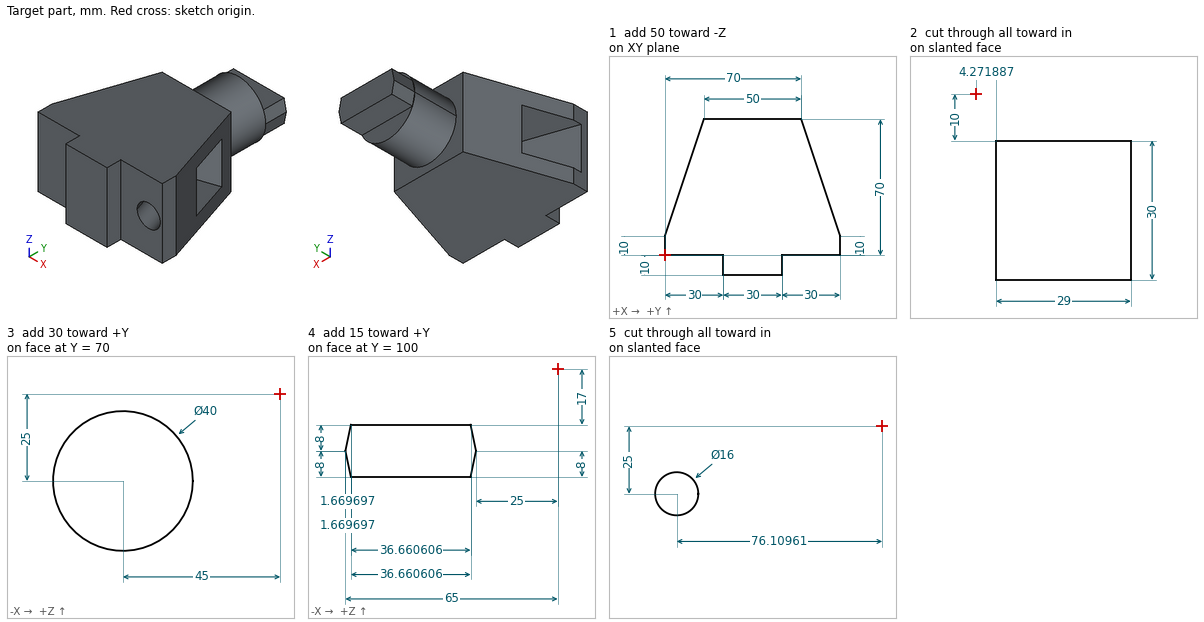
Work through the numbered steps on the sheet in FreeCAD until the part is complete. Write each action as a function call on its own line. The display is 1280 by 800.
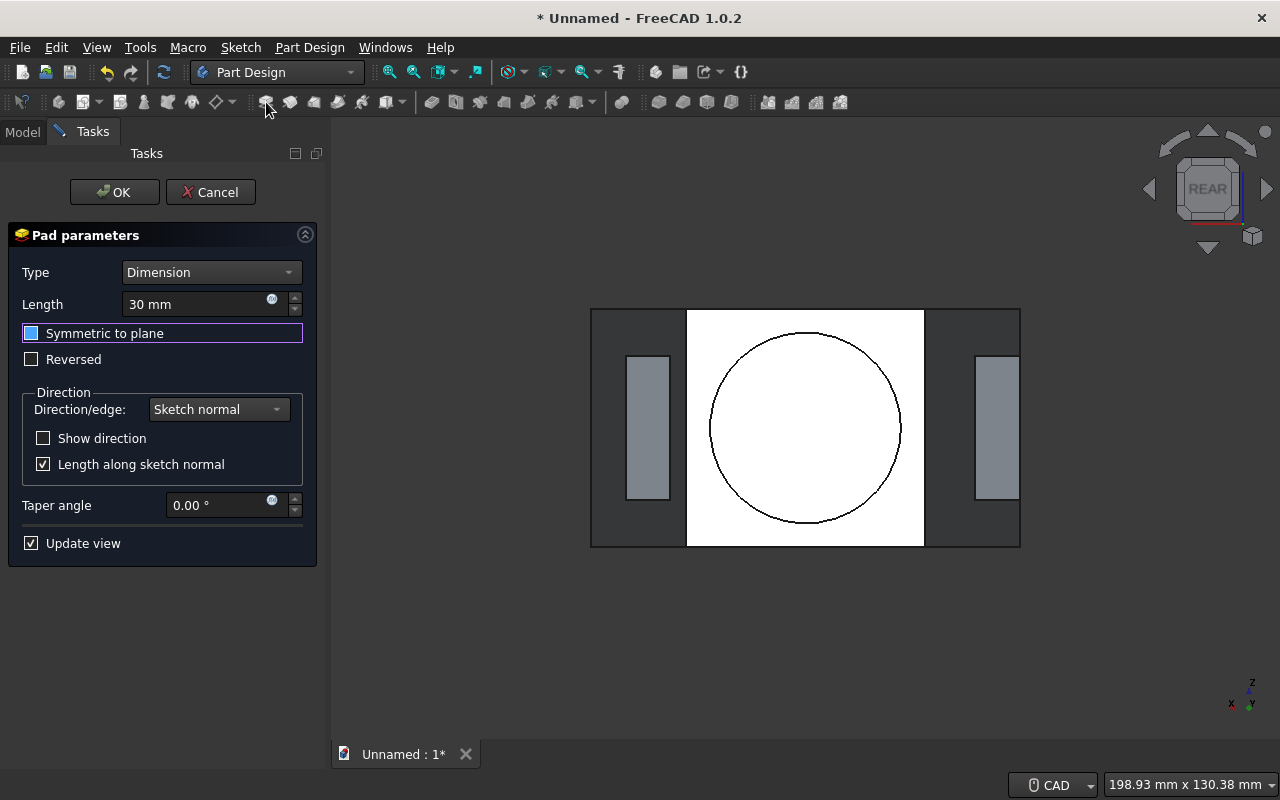
click(115, 192)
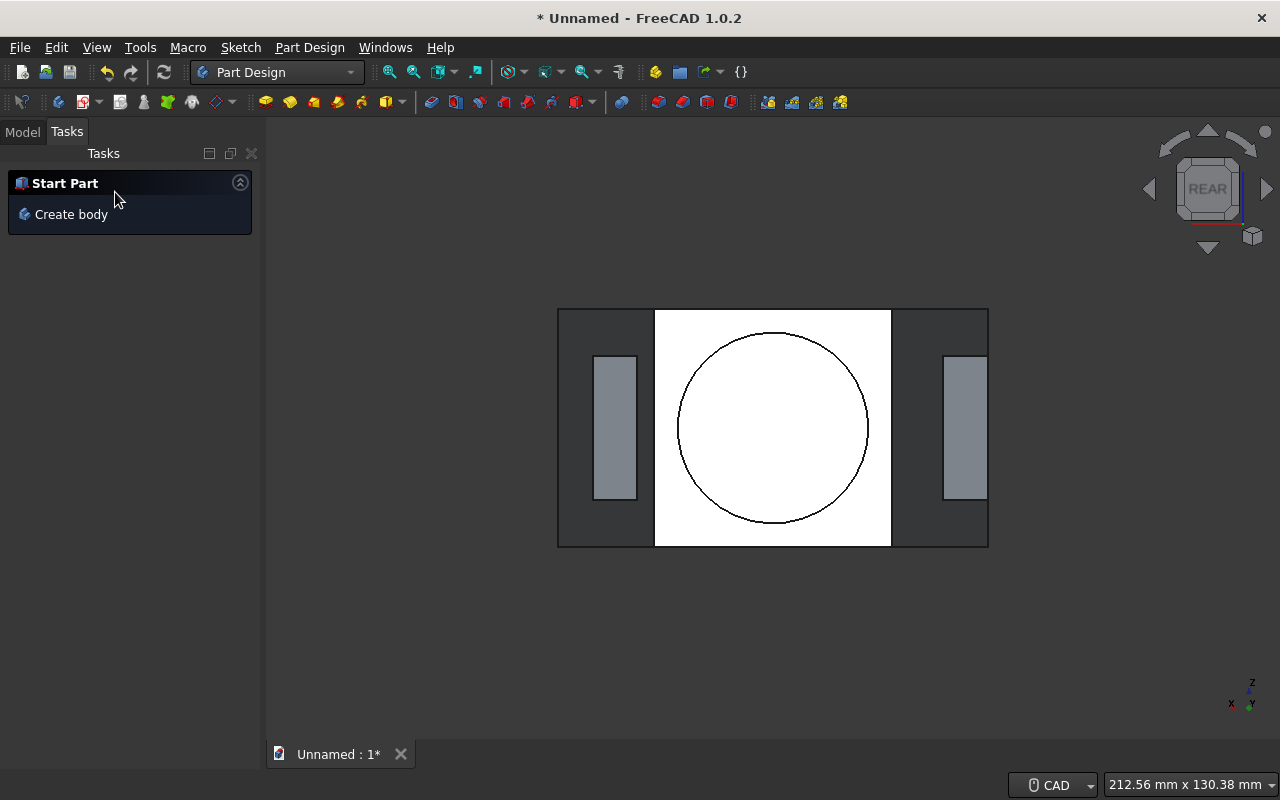
key(v)
key(f)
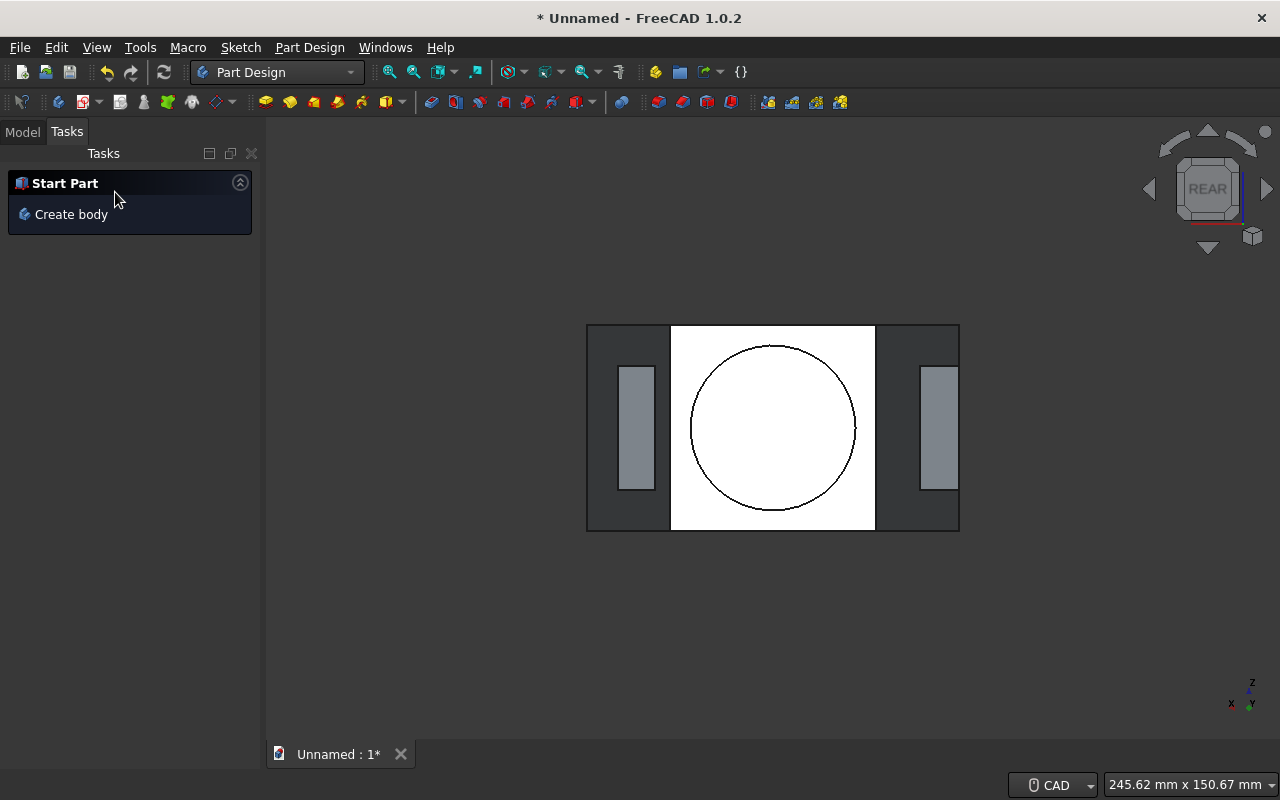
click(773, 427)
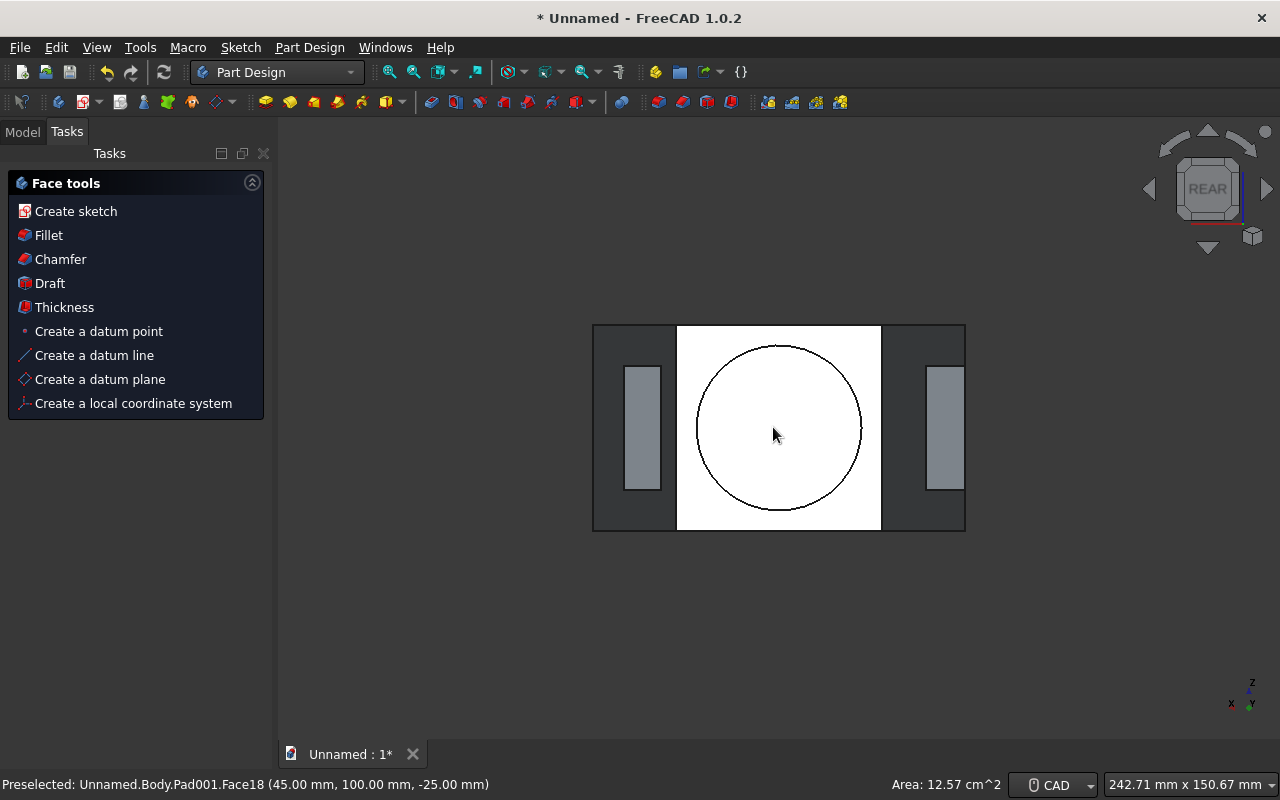
click(84, 102)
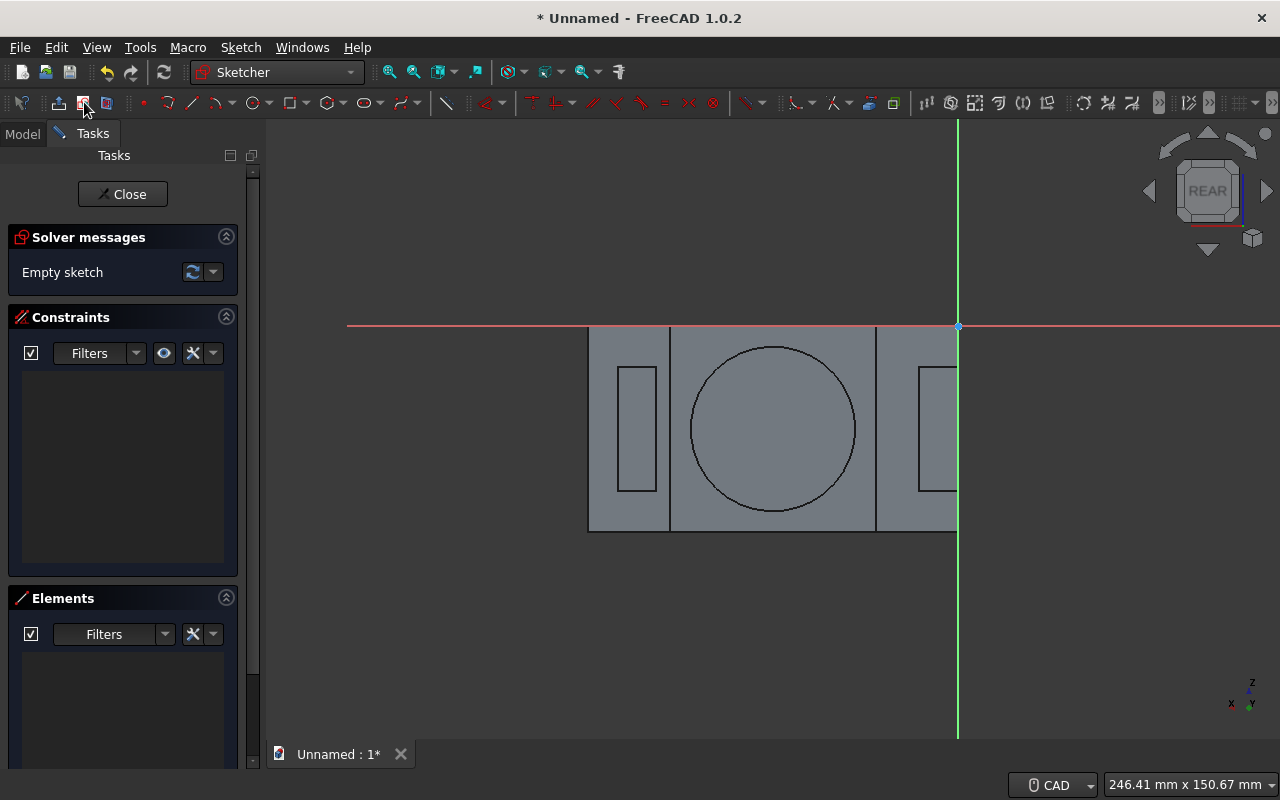
scroll(922, 365, up, 4)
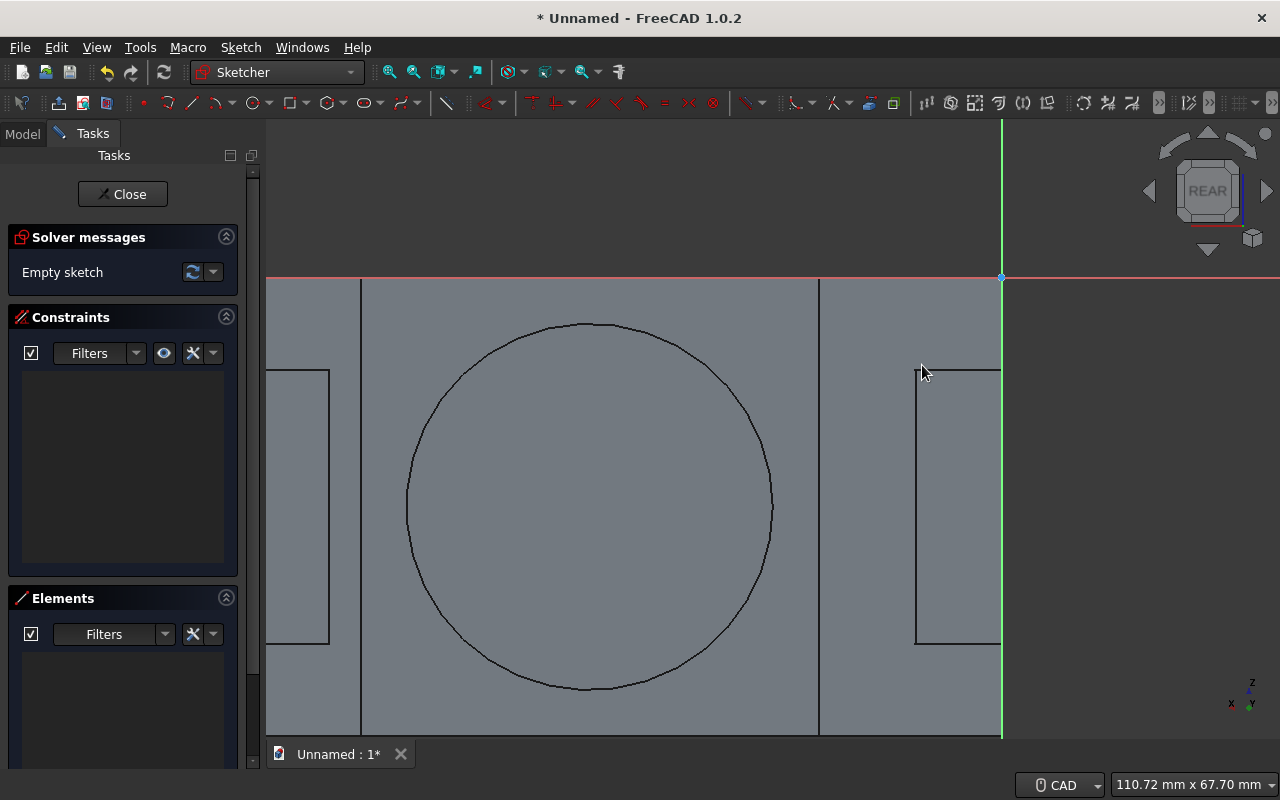
key(g)
key(m)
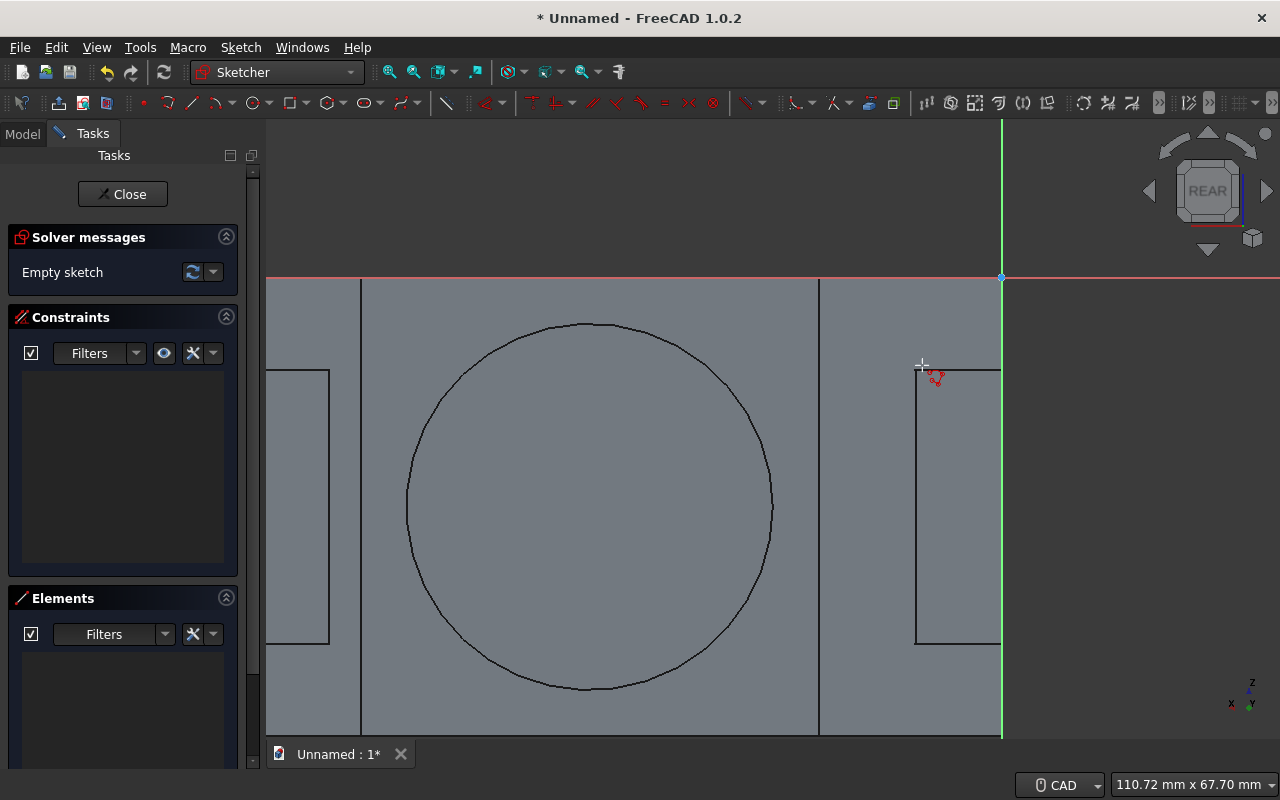
click(757, 434)
click(422, 434)
click(406, 507)
click(422, 580)
click(757, 580)
click(773, 507)
click(757, 435)
key(Escape)
key(Escape)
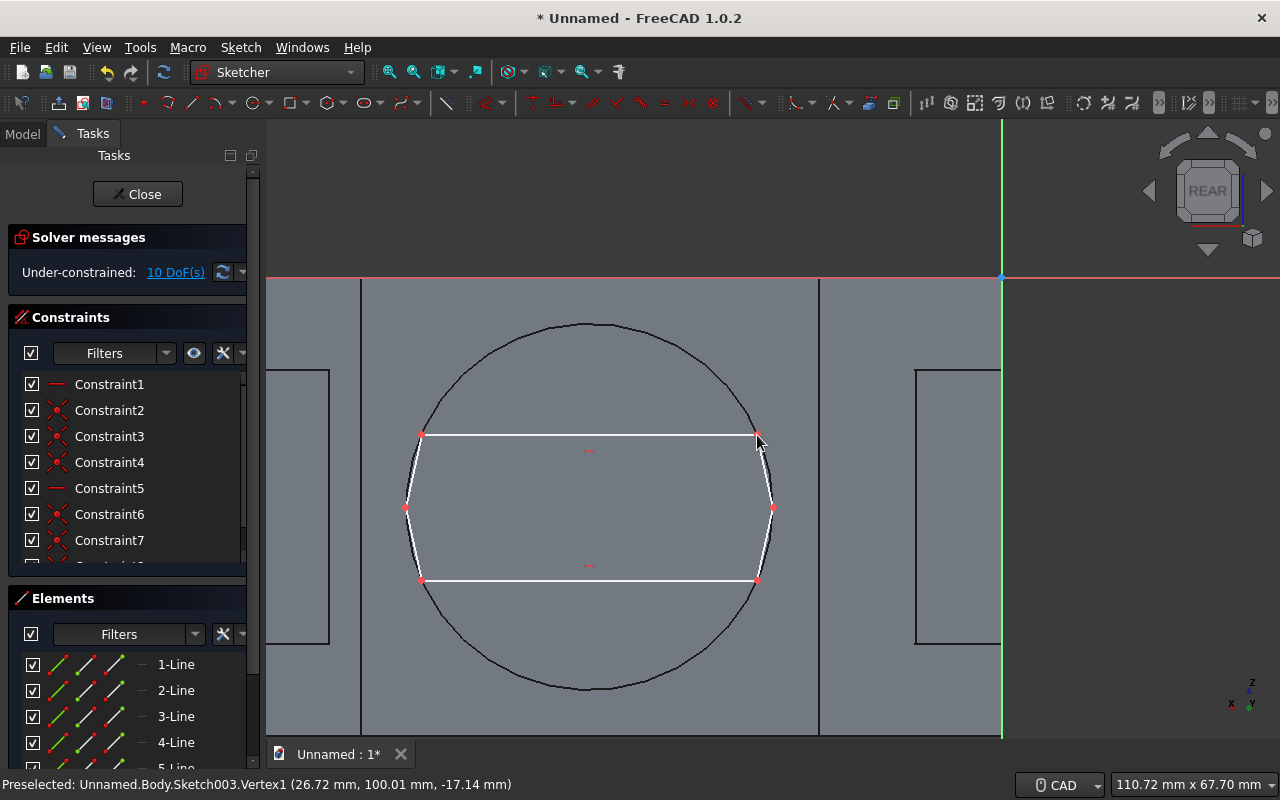
key(d)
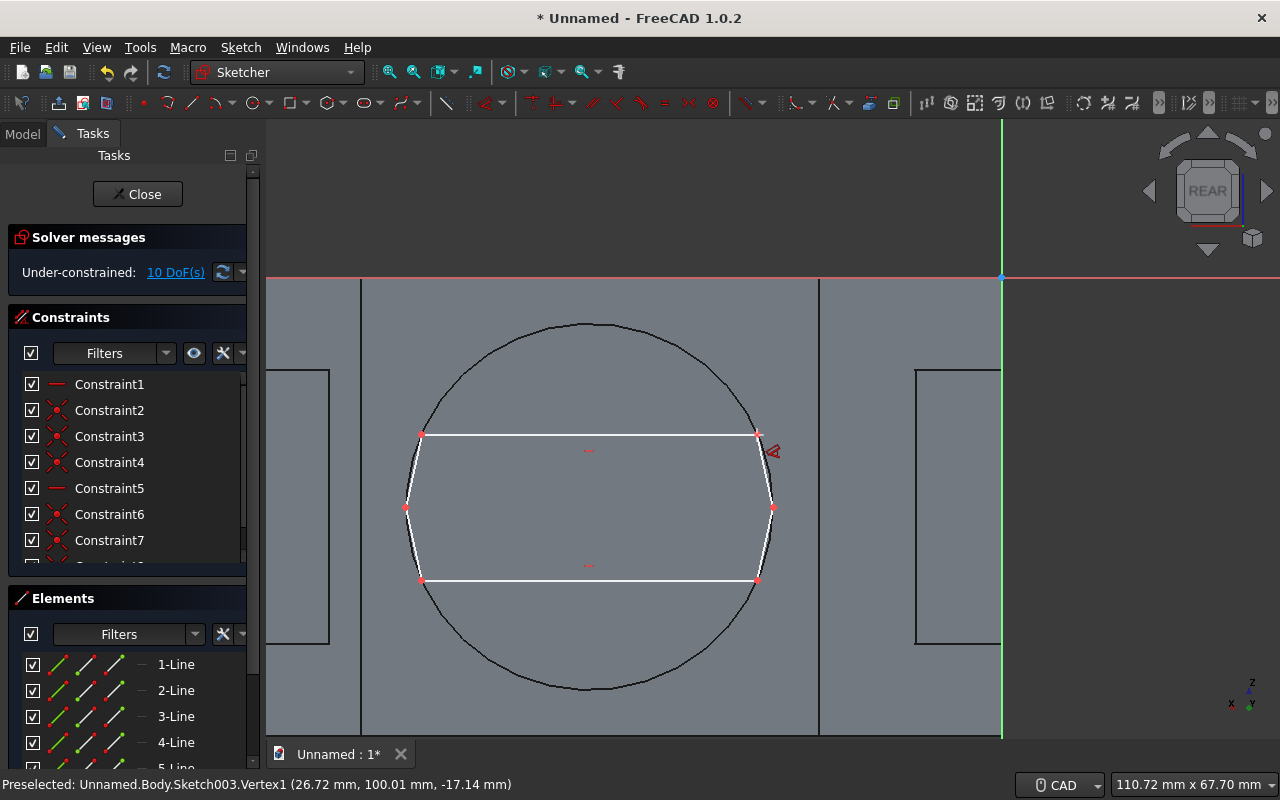
click(417, 457)
click(372, 471)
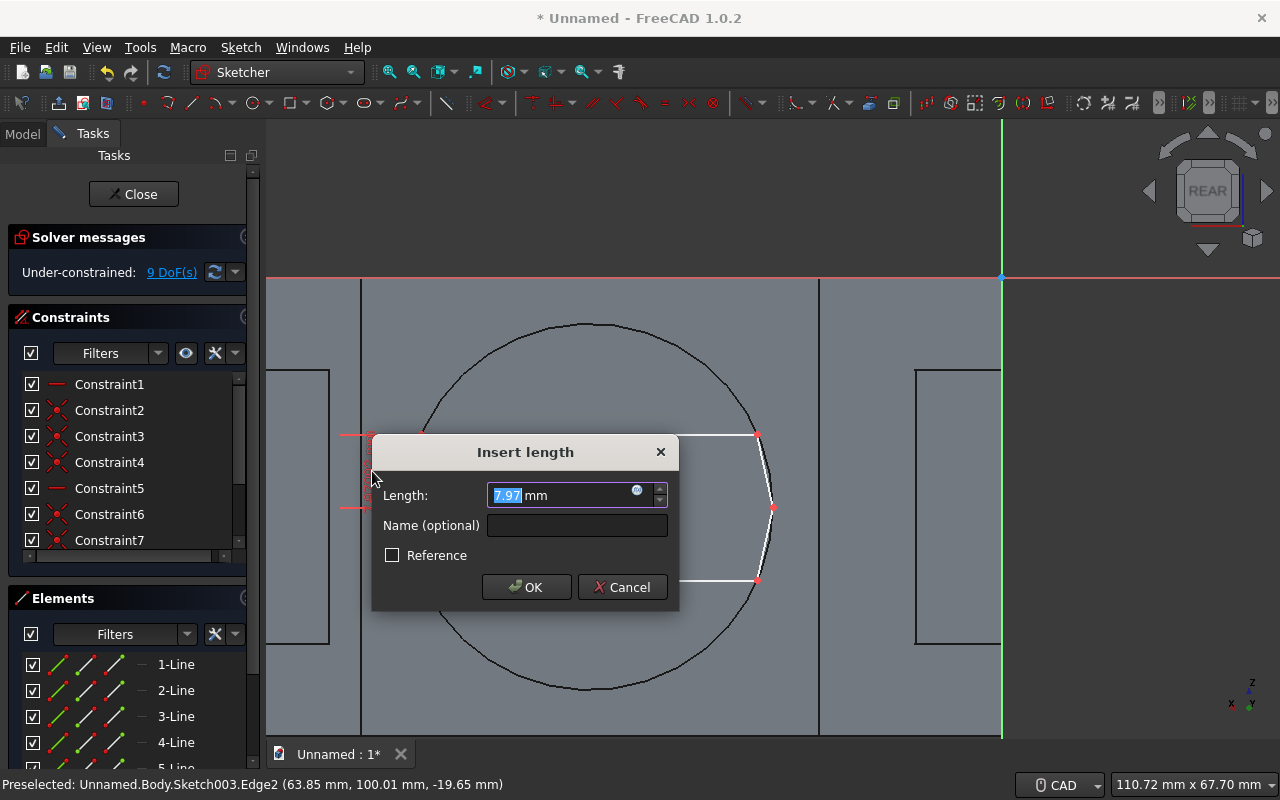
text(8)
key(Return)